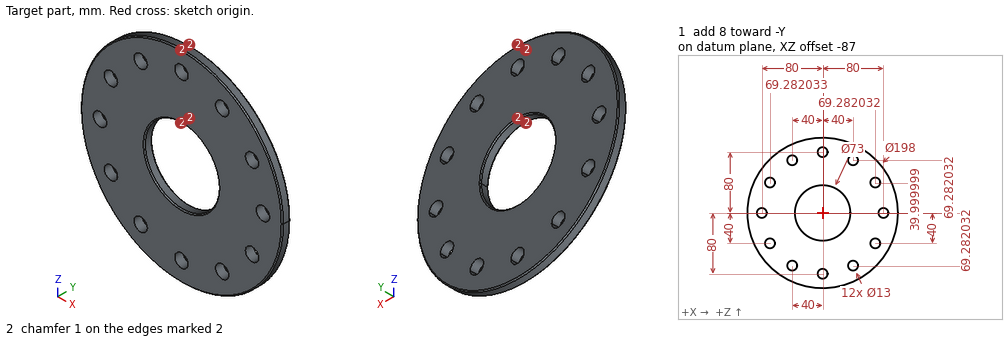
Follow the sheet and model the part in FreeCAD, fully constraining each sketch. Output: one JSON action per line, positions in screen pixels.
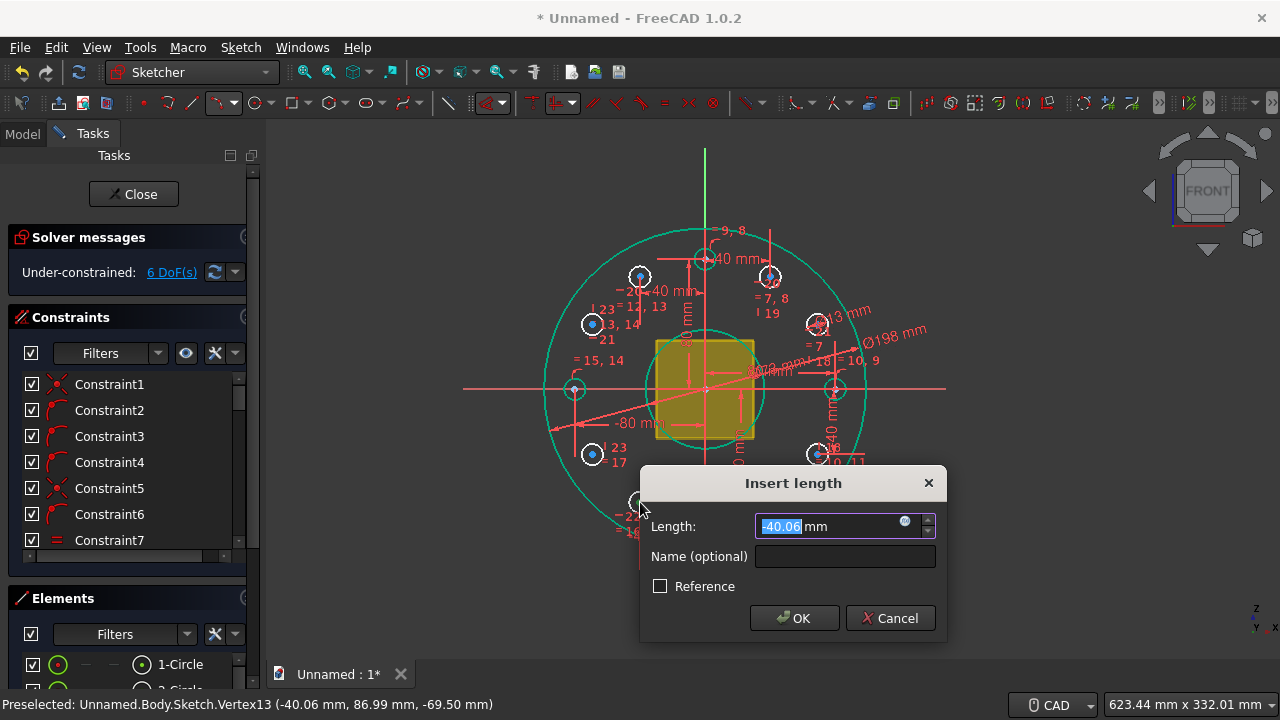
{"action": "type", "text": "-40"}
{"action": "key", "text": "Return"}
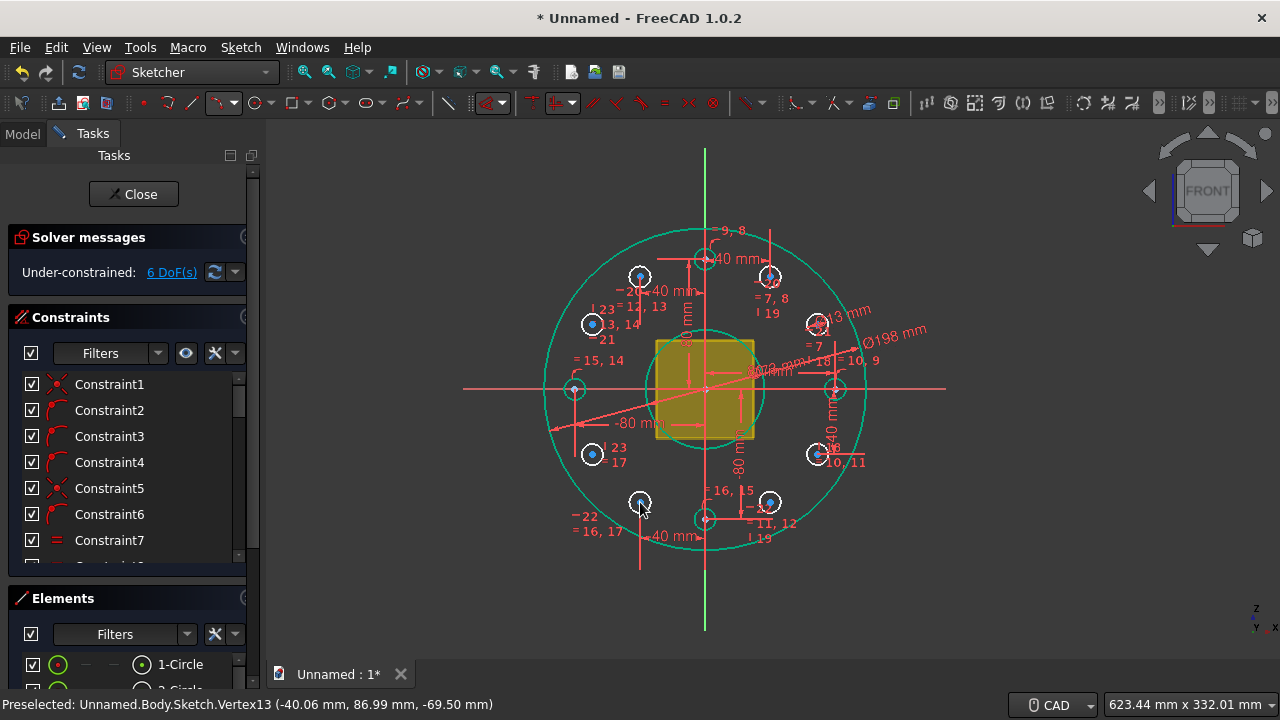
{"action": "left_click", "coordinate": [592, 455]}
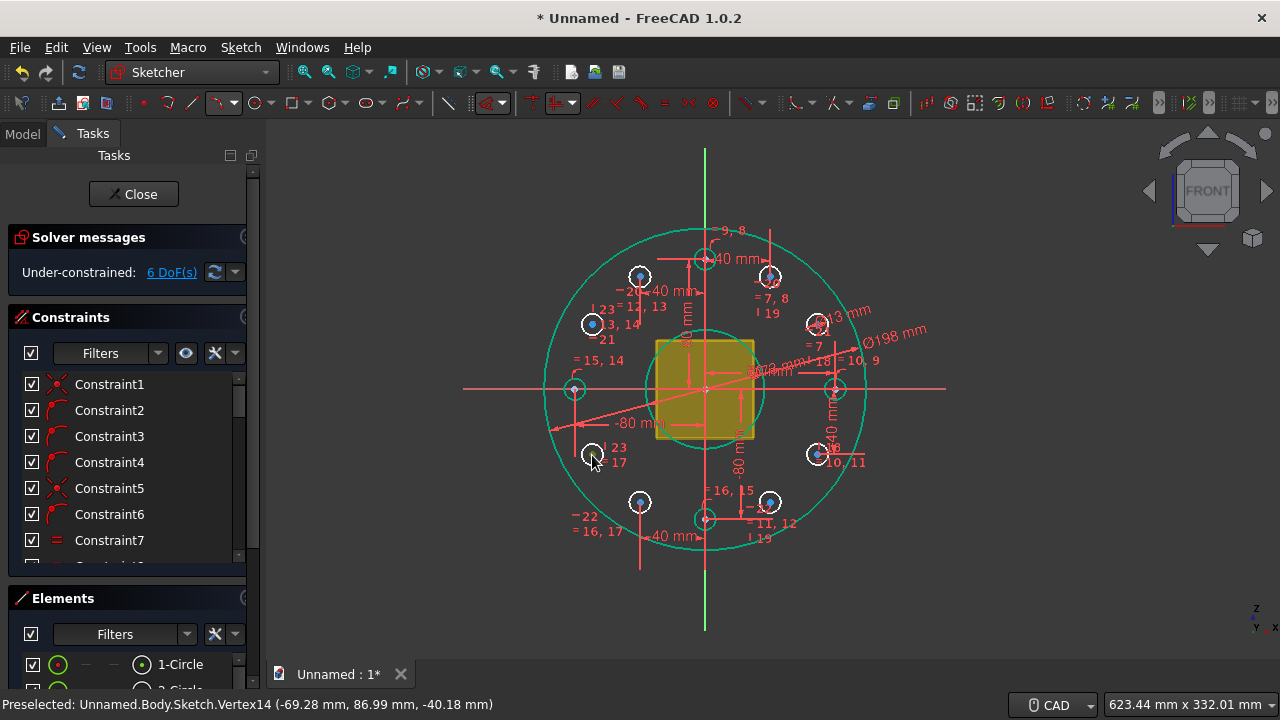
{"action": "key", "text": "i"}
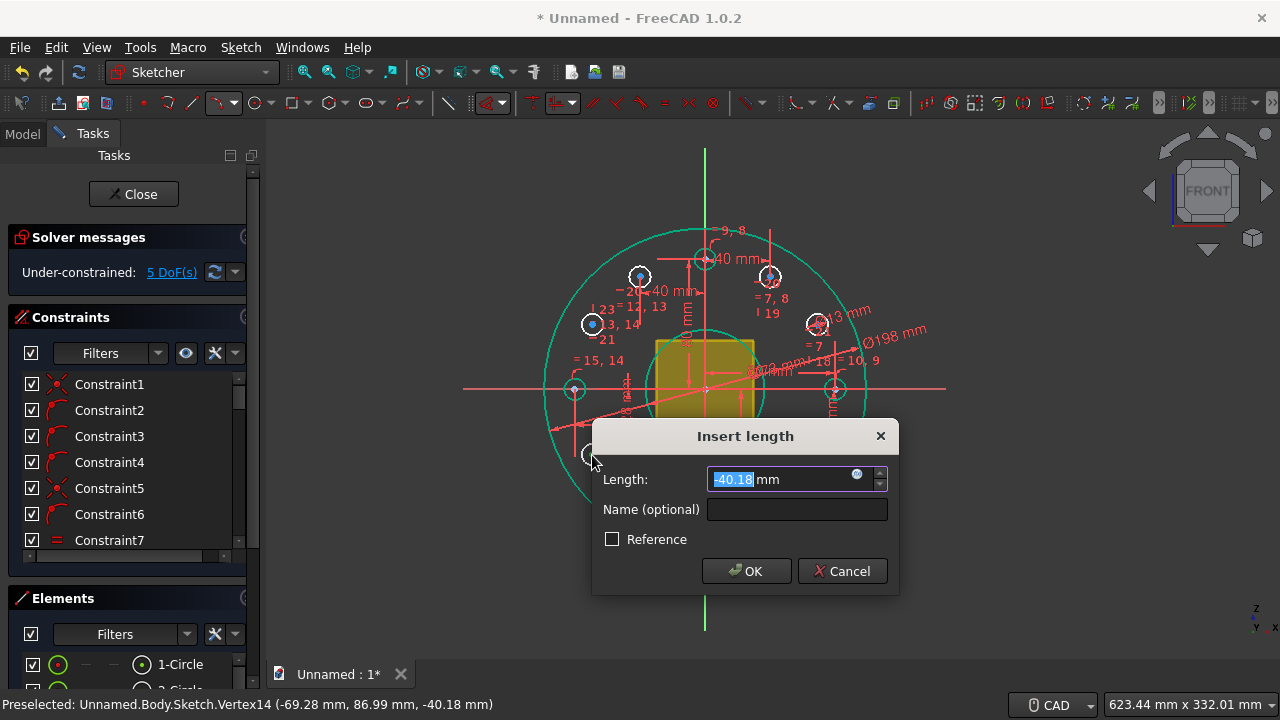
{"action": "type", "text": "-40"}
{"action": "key", "text": "Return"}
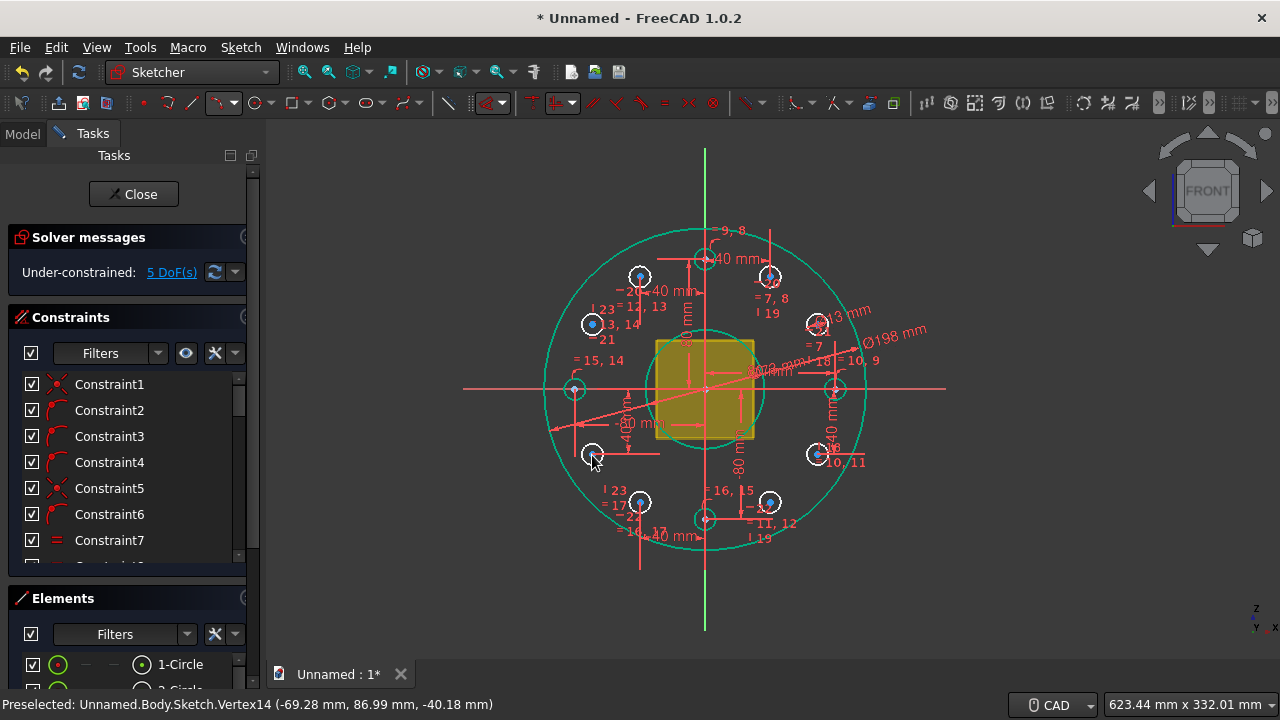
{"action": "left_click", "coordinate": [818, 325]}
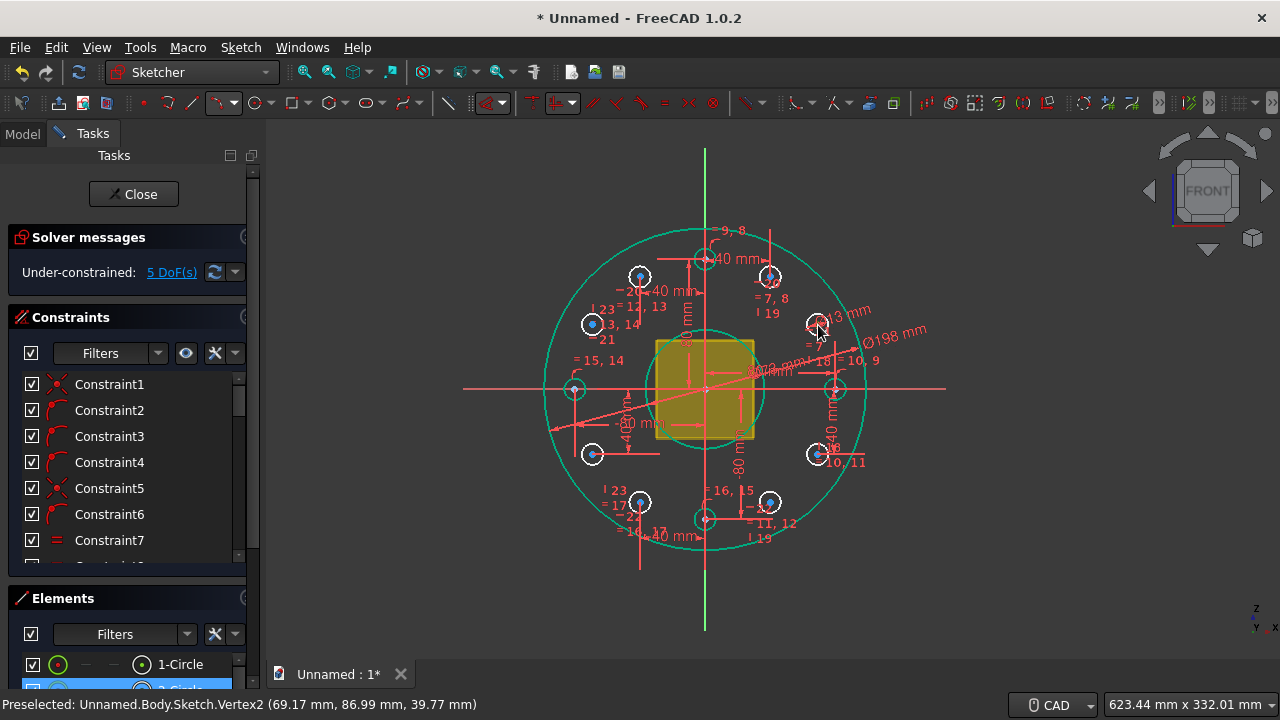
{"action": "key", "text": "l"}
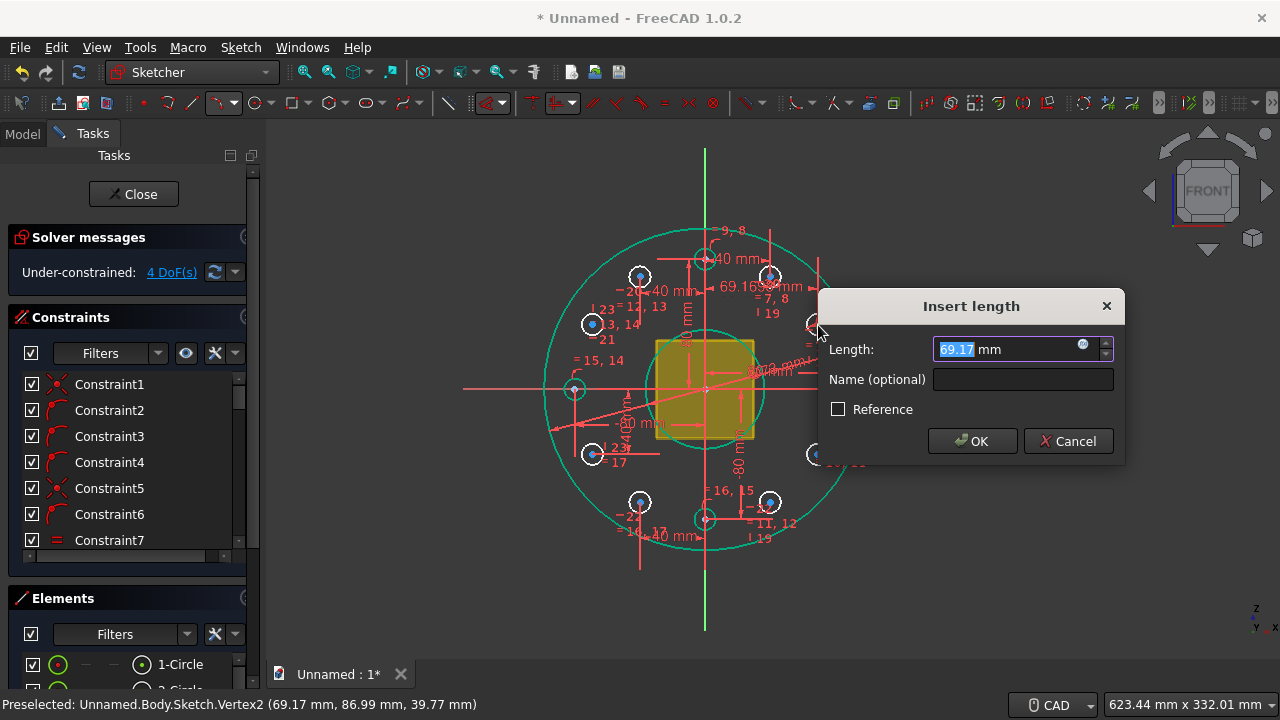
{"action": "type", "text": "69.282032"}
{"action": "key", "text": "Return"}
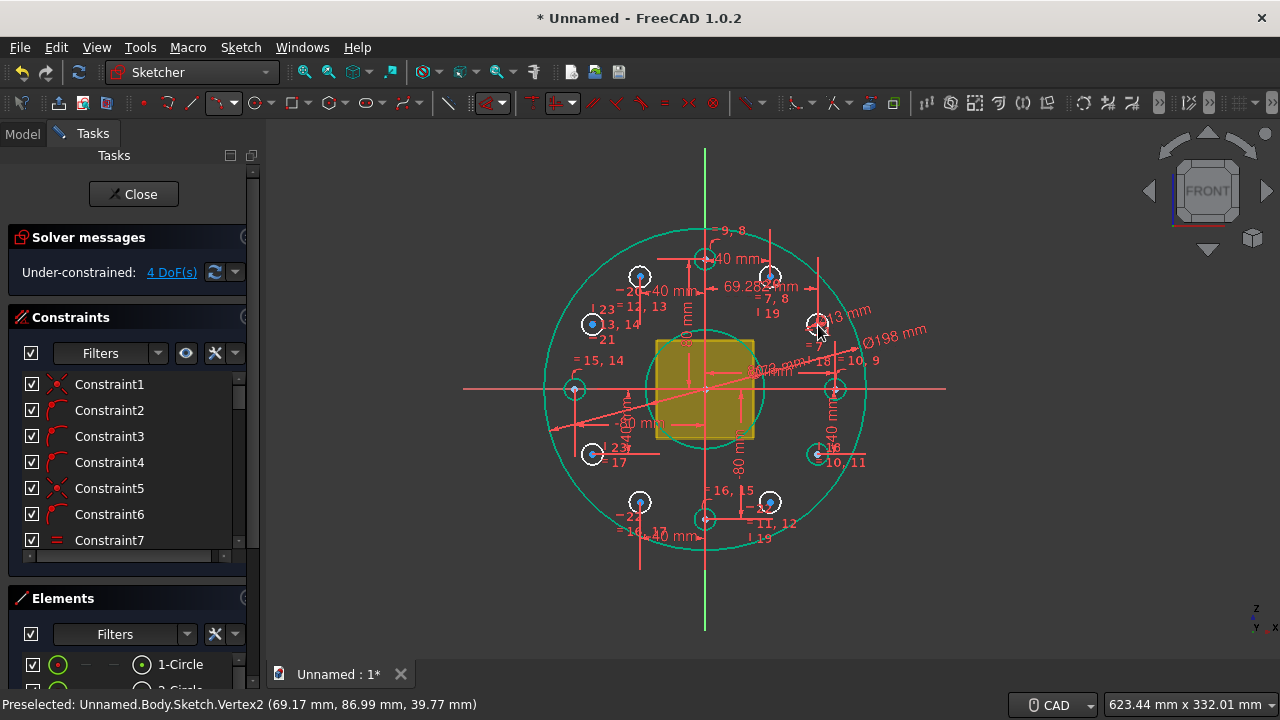
{"action": "left_click", "coordinate": [818, 325]}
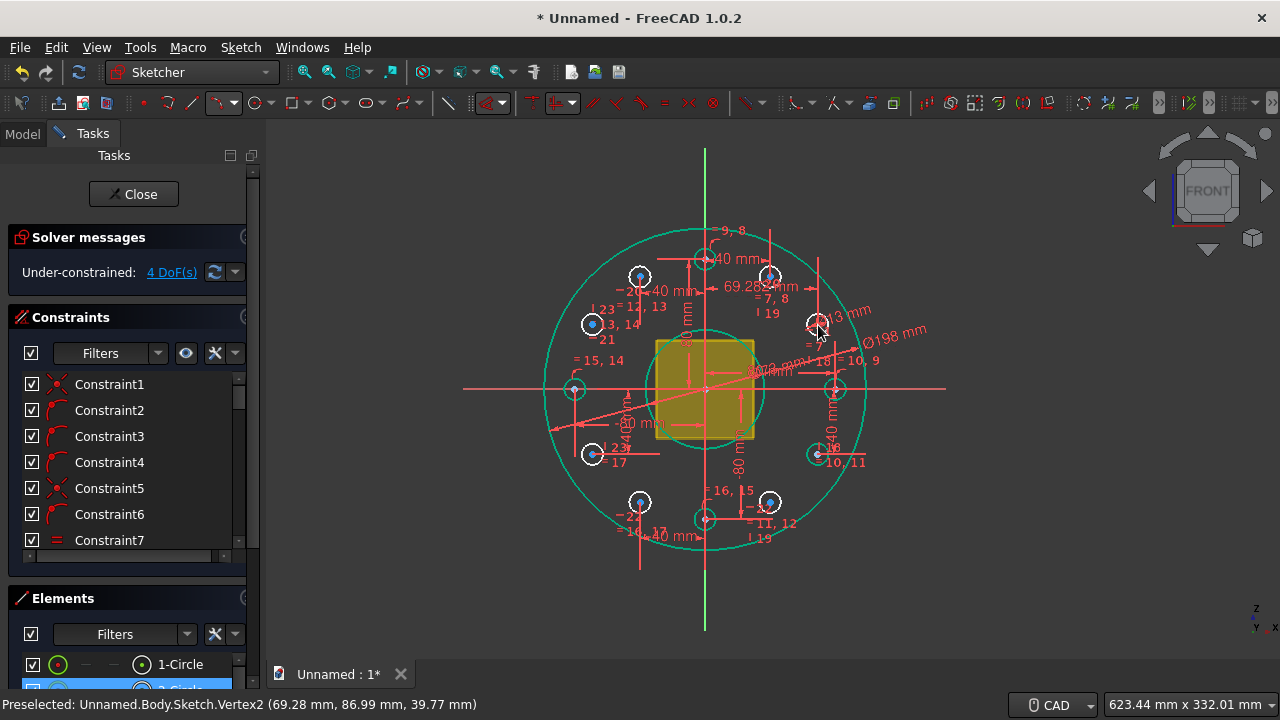
{"action": "key", "text": "i"}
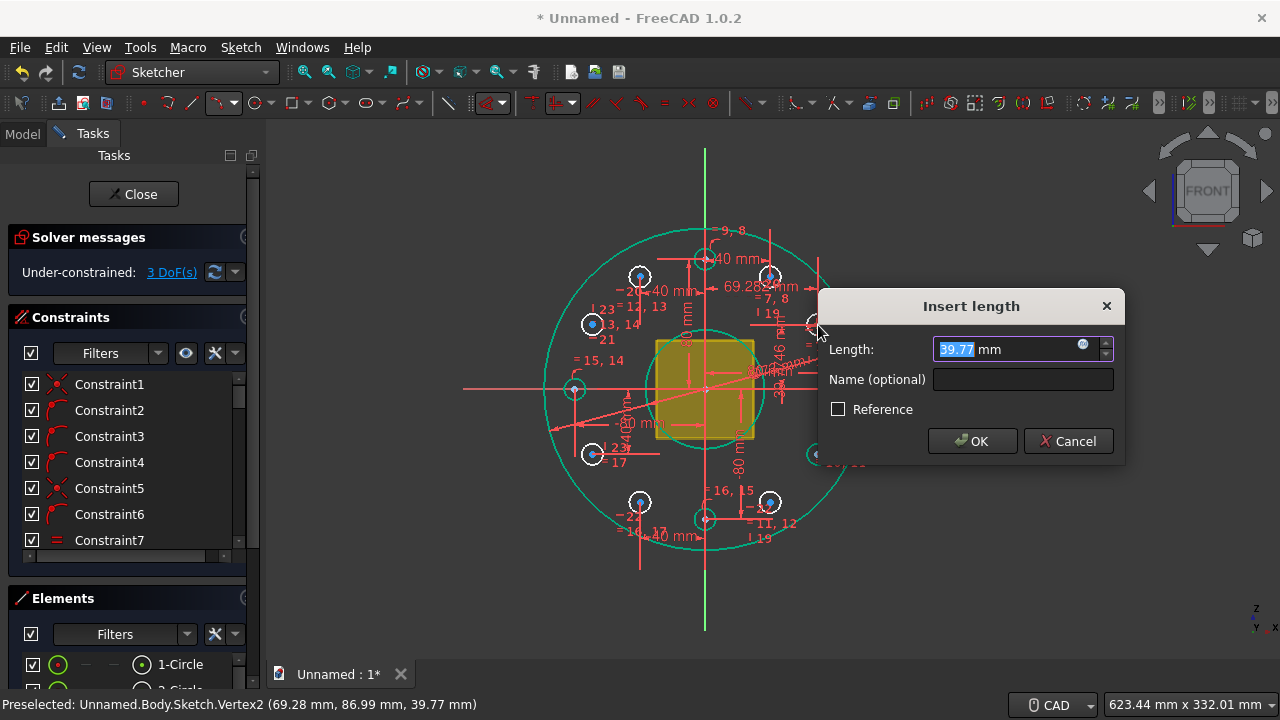
{"action": "type", "text": "39.999999"}
{"action": "key", "text": "Return"}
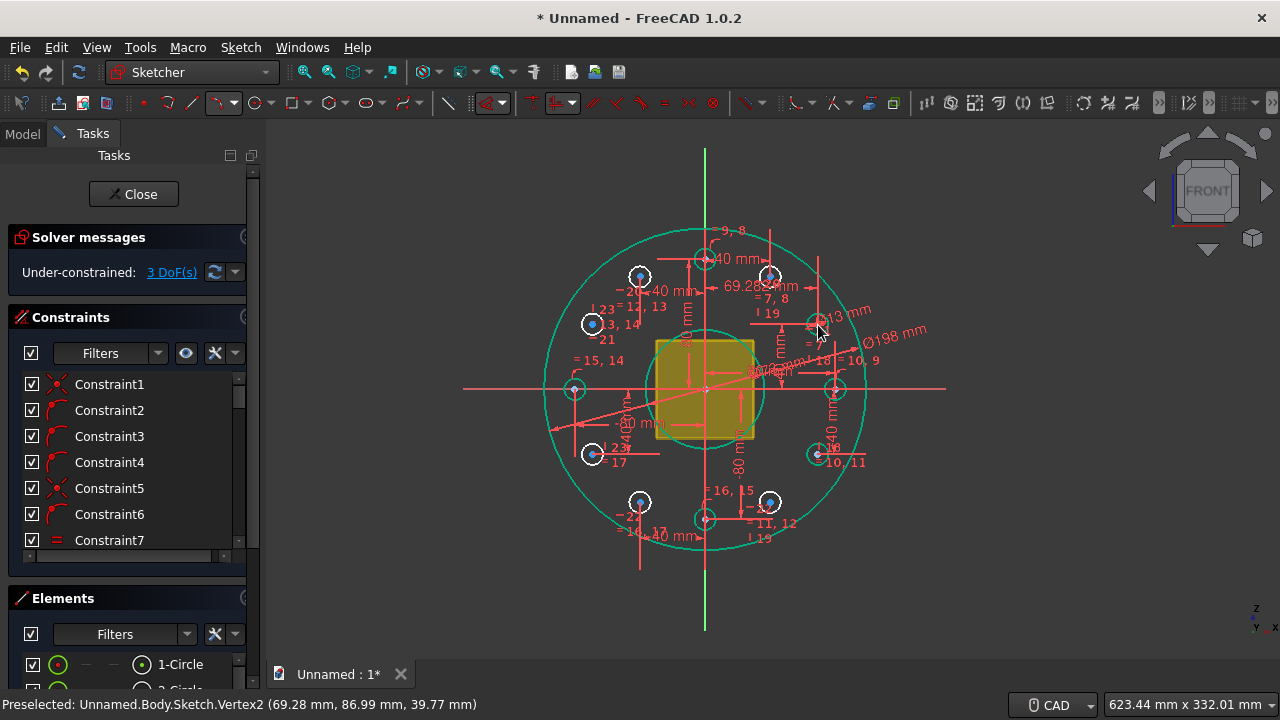
{"action": "left_click", "coordinate": [770, 277]}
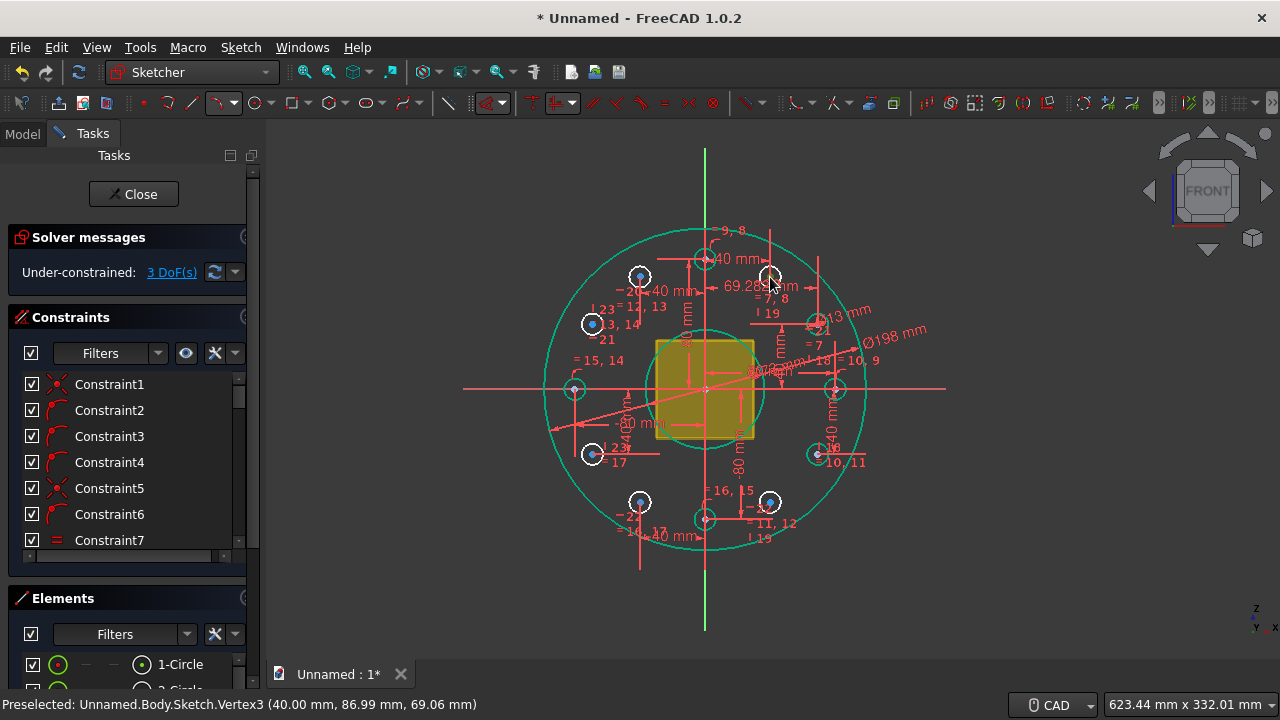
{"action": "left_click", "coordinate": [504, 104]}